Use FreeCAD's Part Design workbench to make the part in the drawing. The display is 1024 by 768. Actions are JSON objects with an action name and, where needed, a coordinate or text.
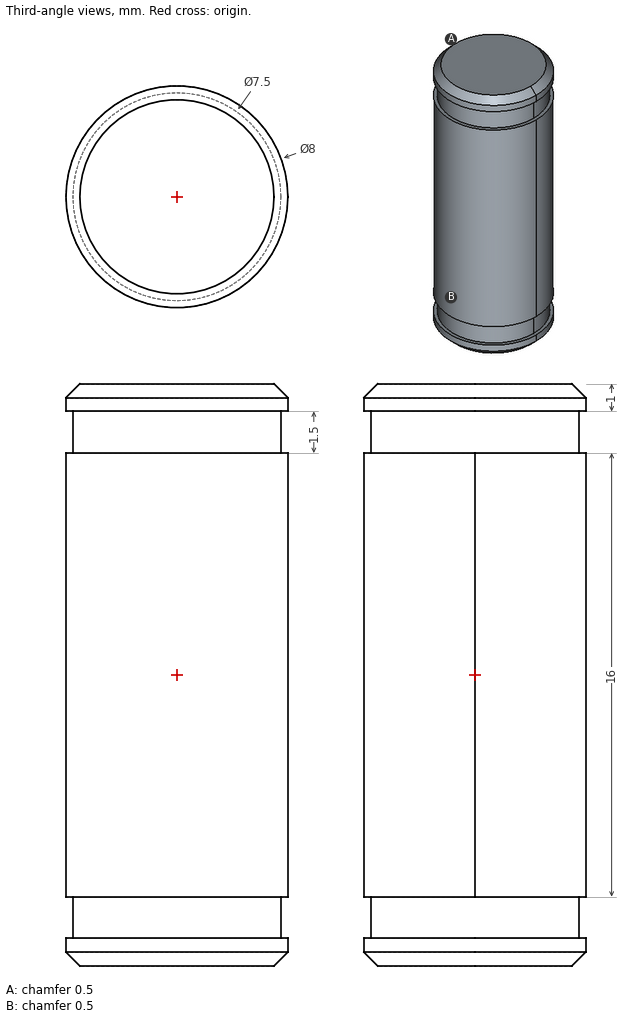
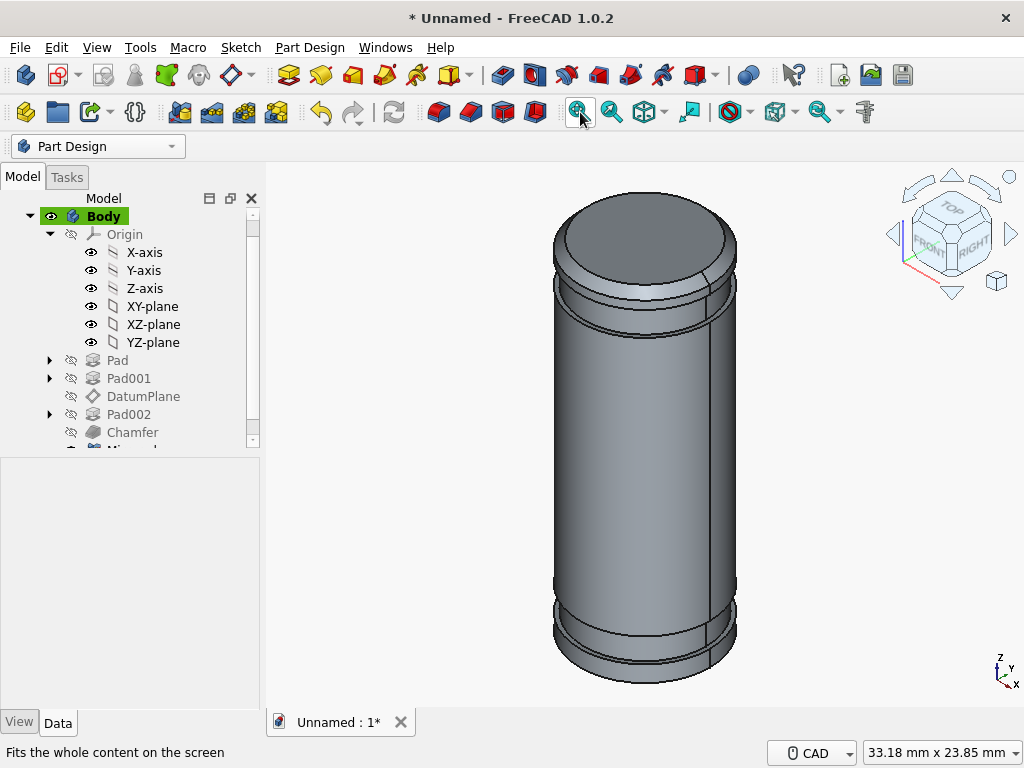
{"action": "left_click", "coordinate": [721, 659]}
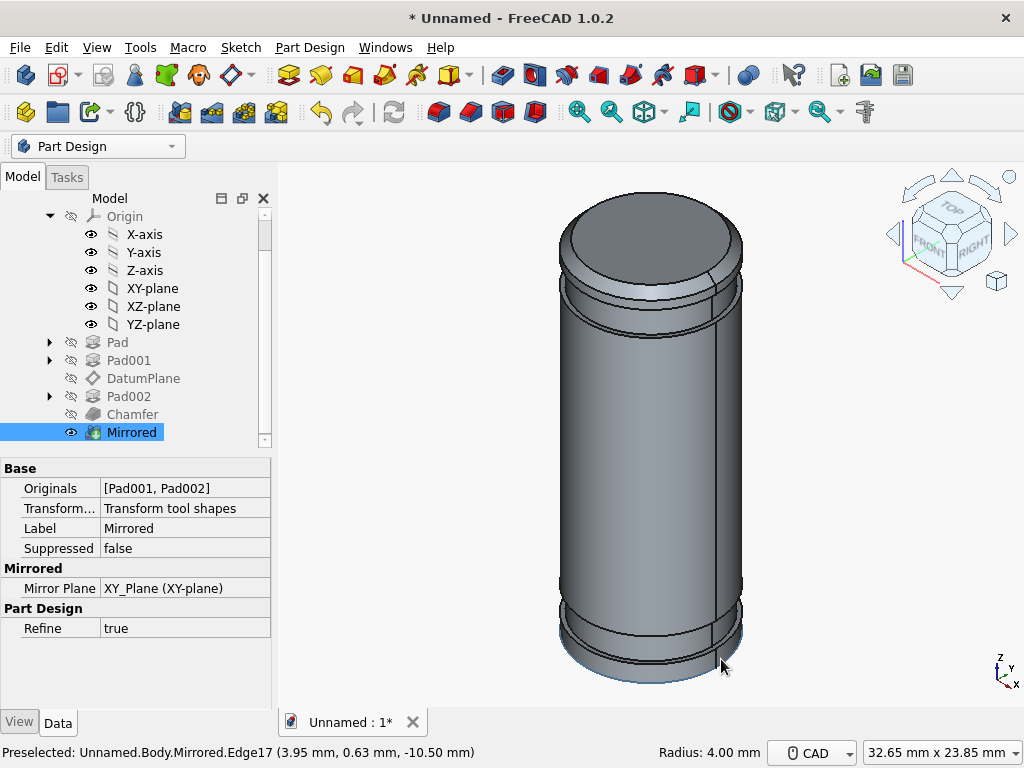
{"action": "left_click", "coordinate": [472, 112]}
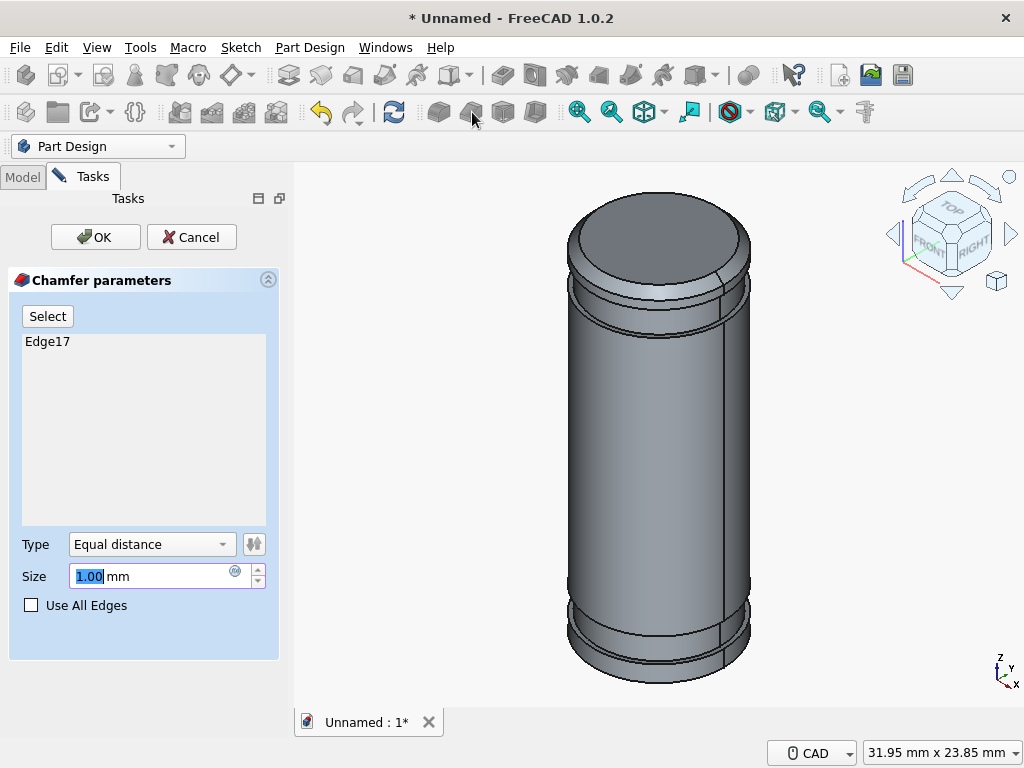
{"action": "type", "text": "0.5"}
{"action": "key", "text": "Tab"}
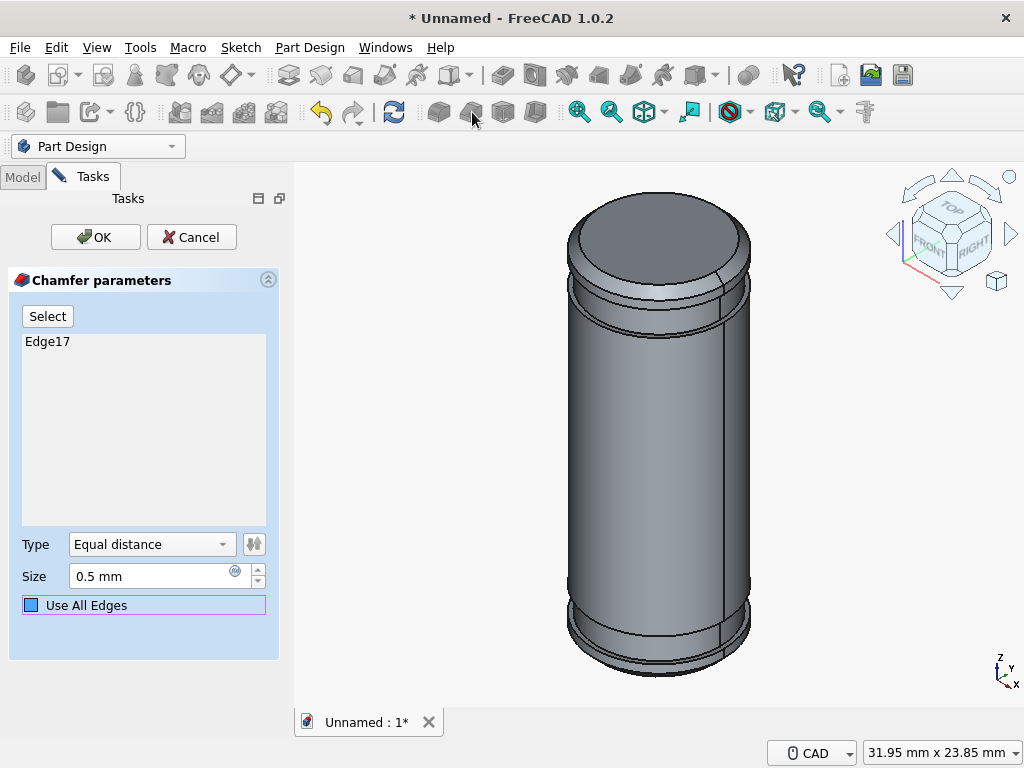
{"action": "left_click", "coordinate": [96, 237]}